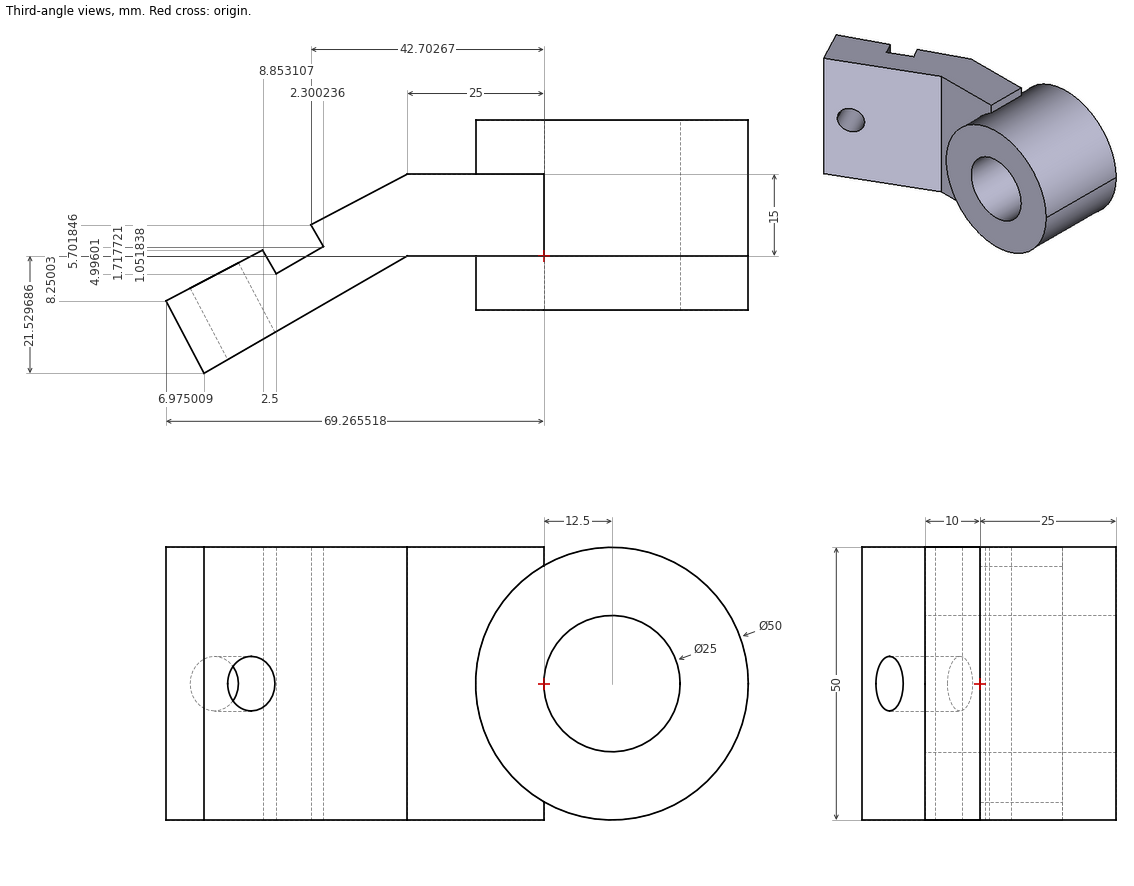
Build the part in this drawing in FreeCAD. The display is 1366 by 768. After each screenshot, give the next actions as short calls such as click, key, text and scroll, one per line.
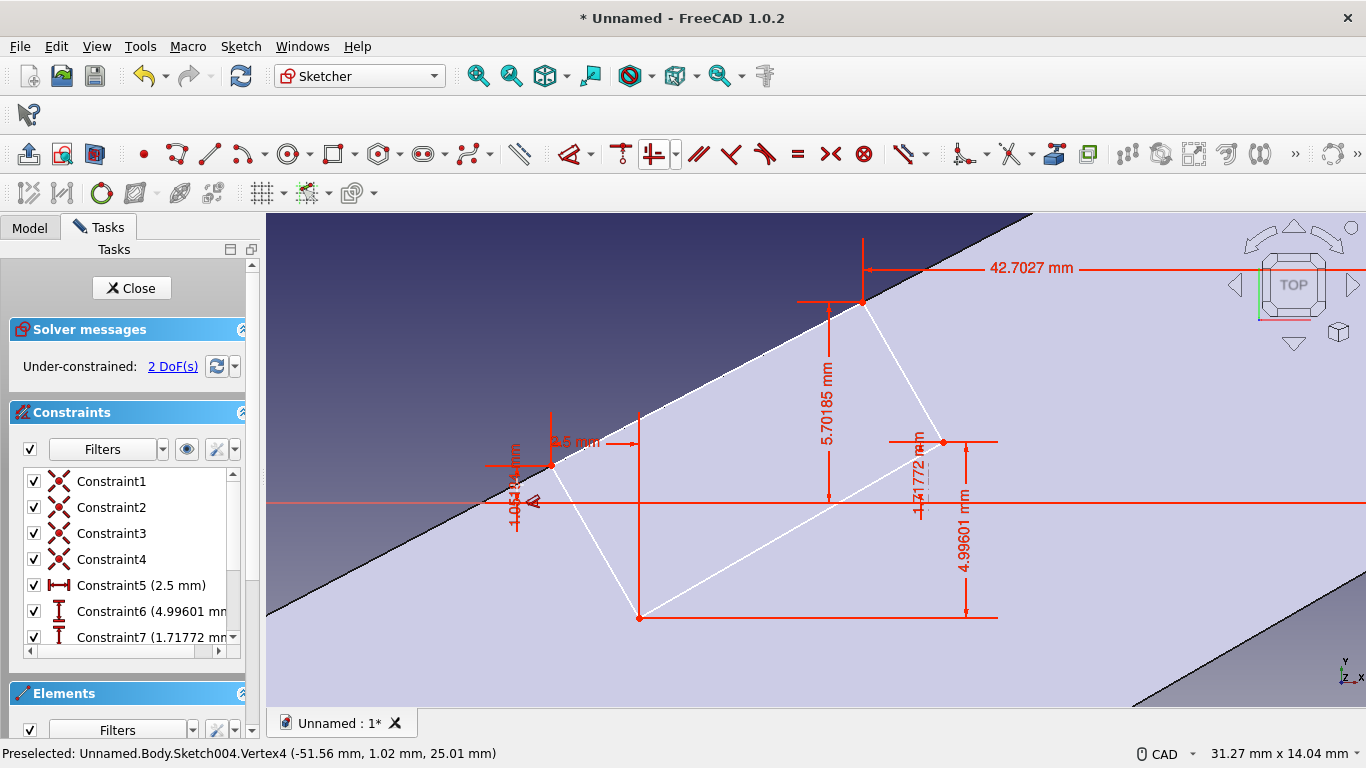
click(919, 400)
click(903, 268)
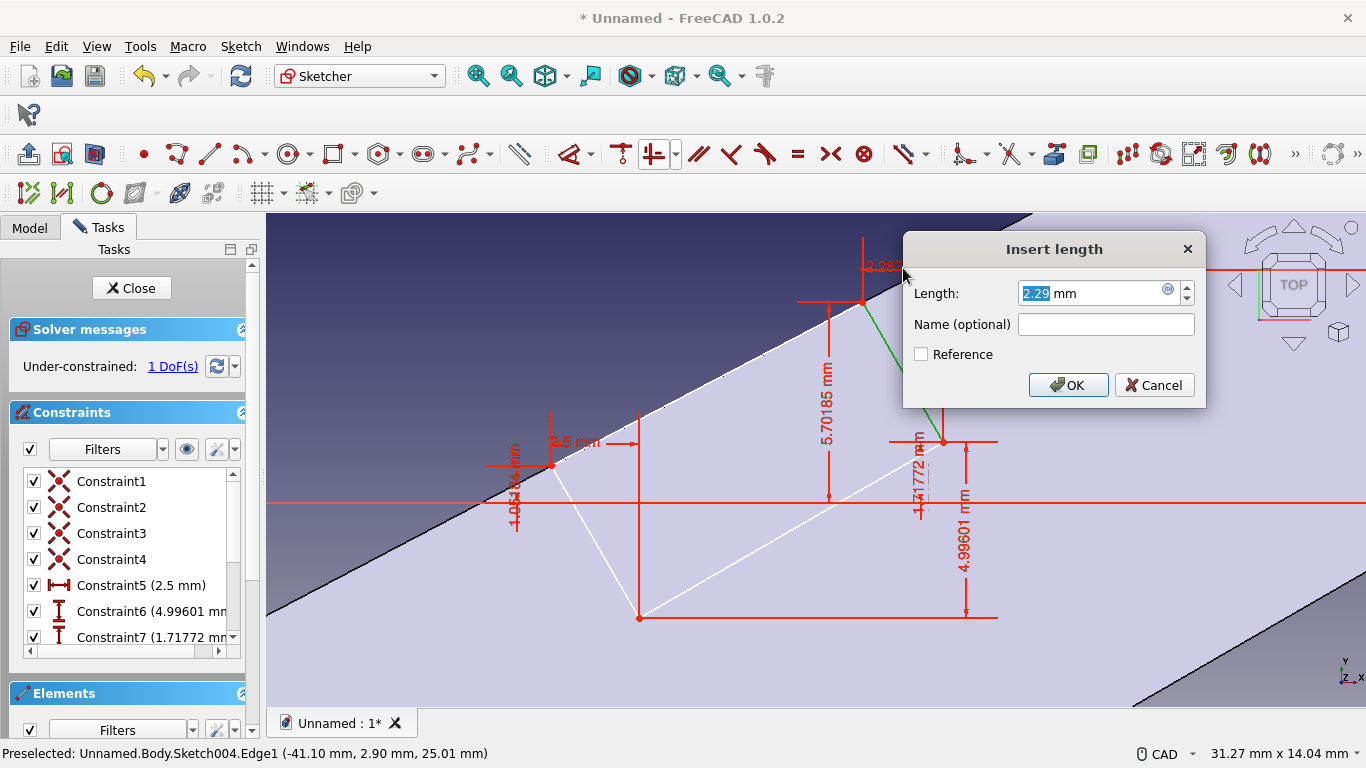
text(2.300236)
key(Return)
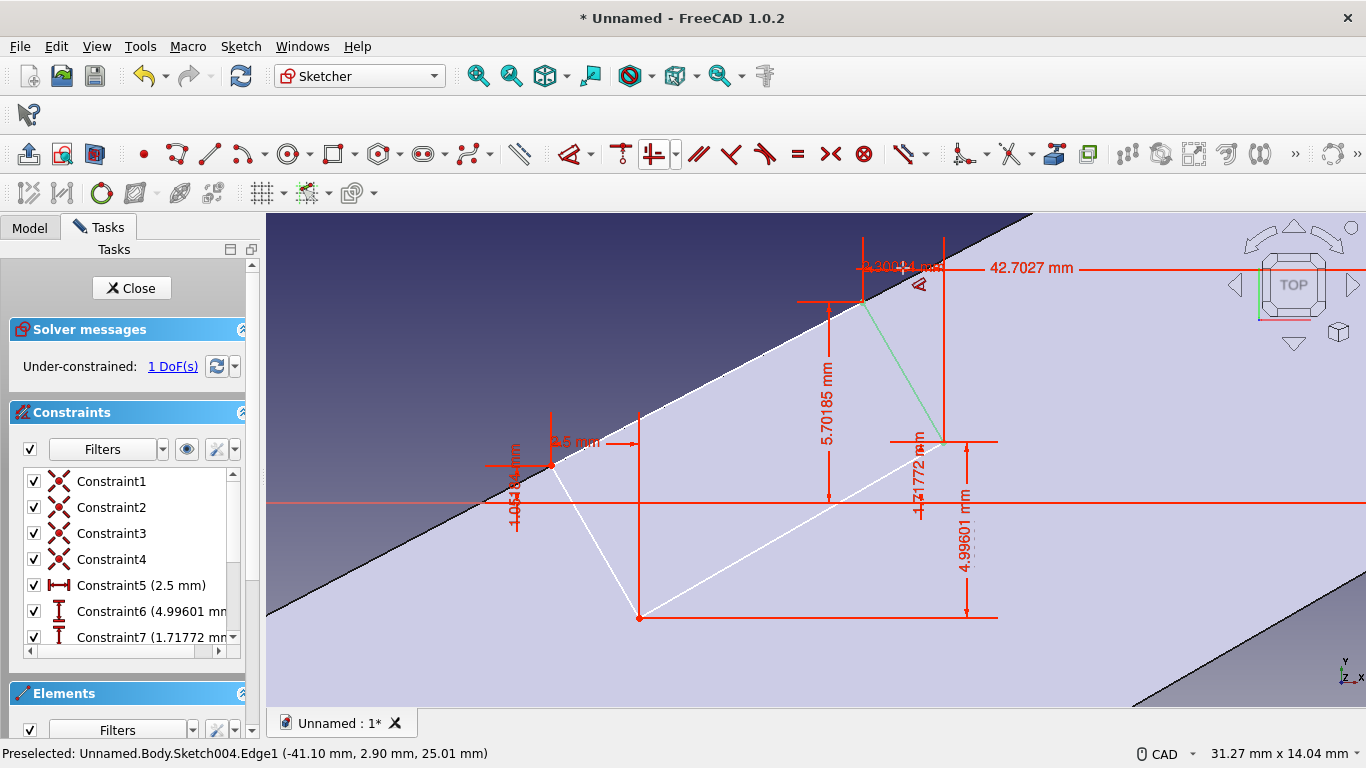
click(769, 351)
click(707, 268)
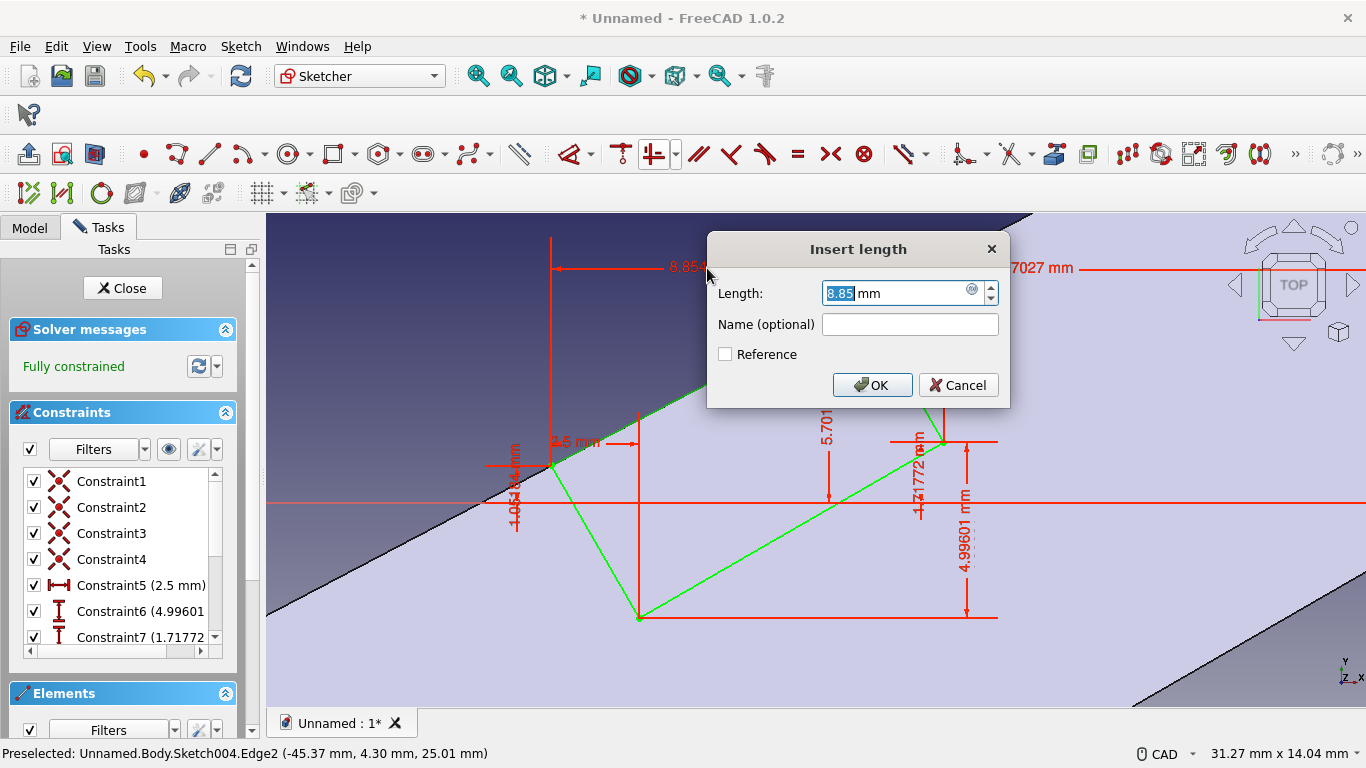
text(8.853107)
key(Return)
key(Escape)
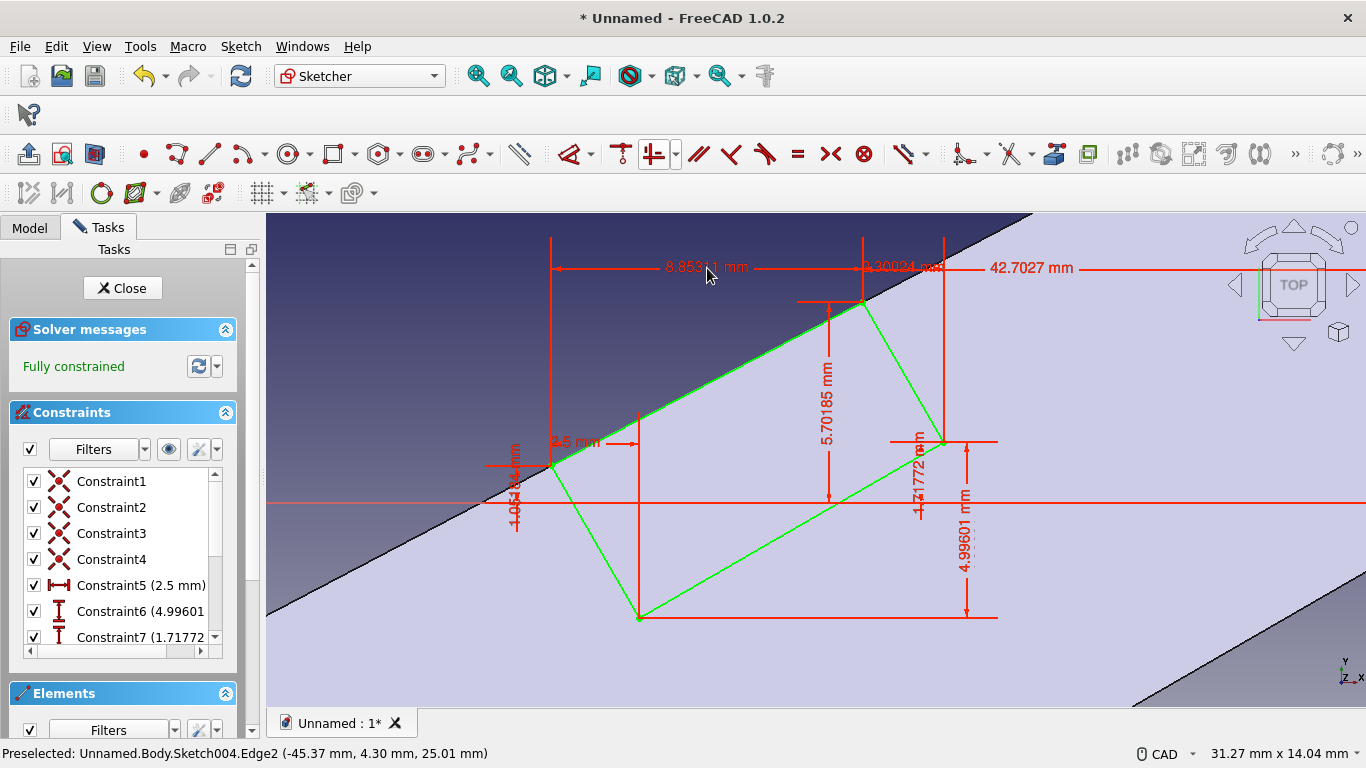
click(123, 288)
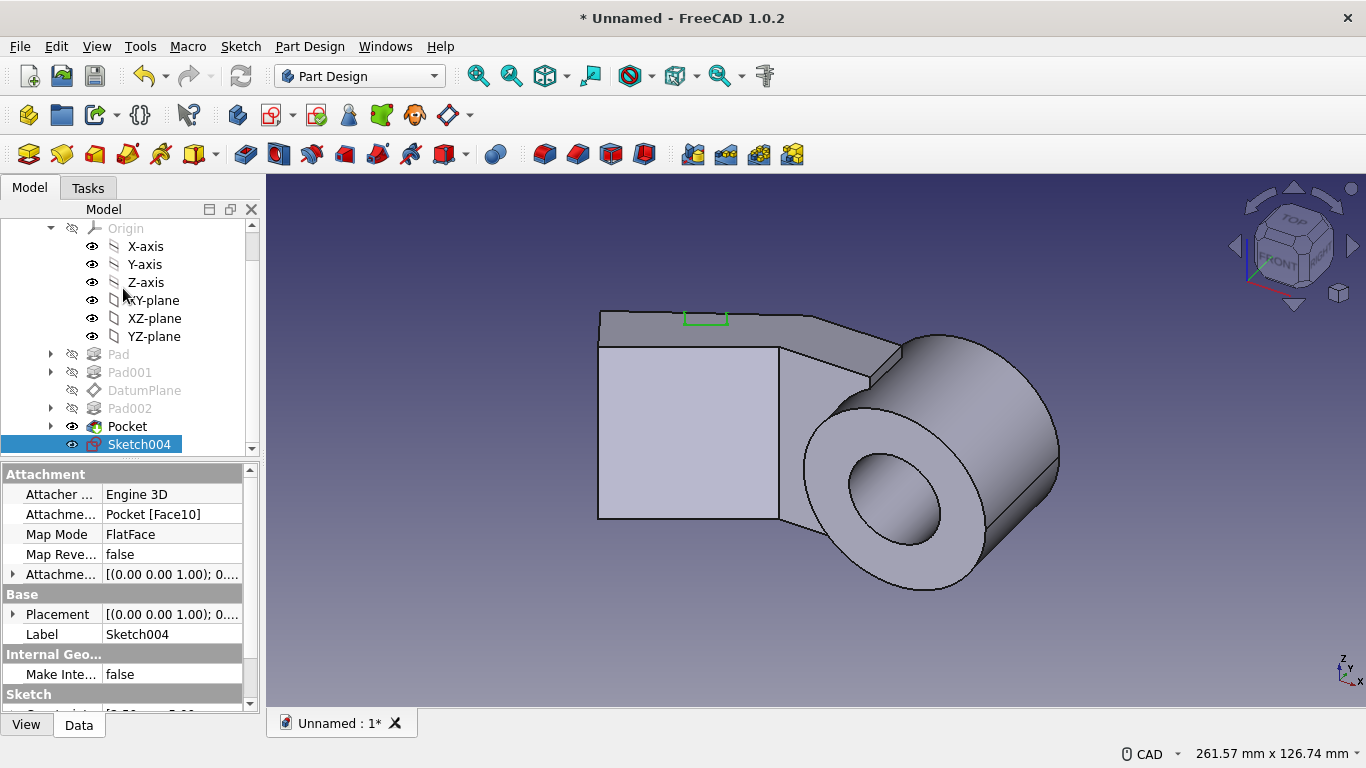
click(246, 154)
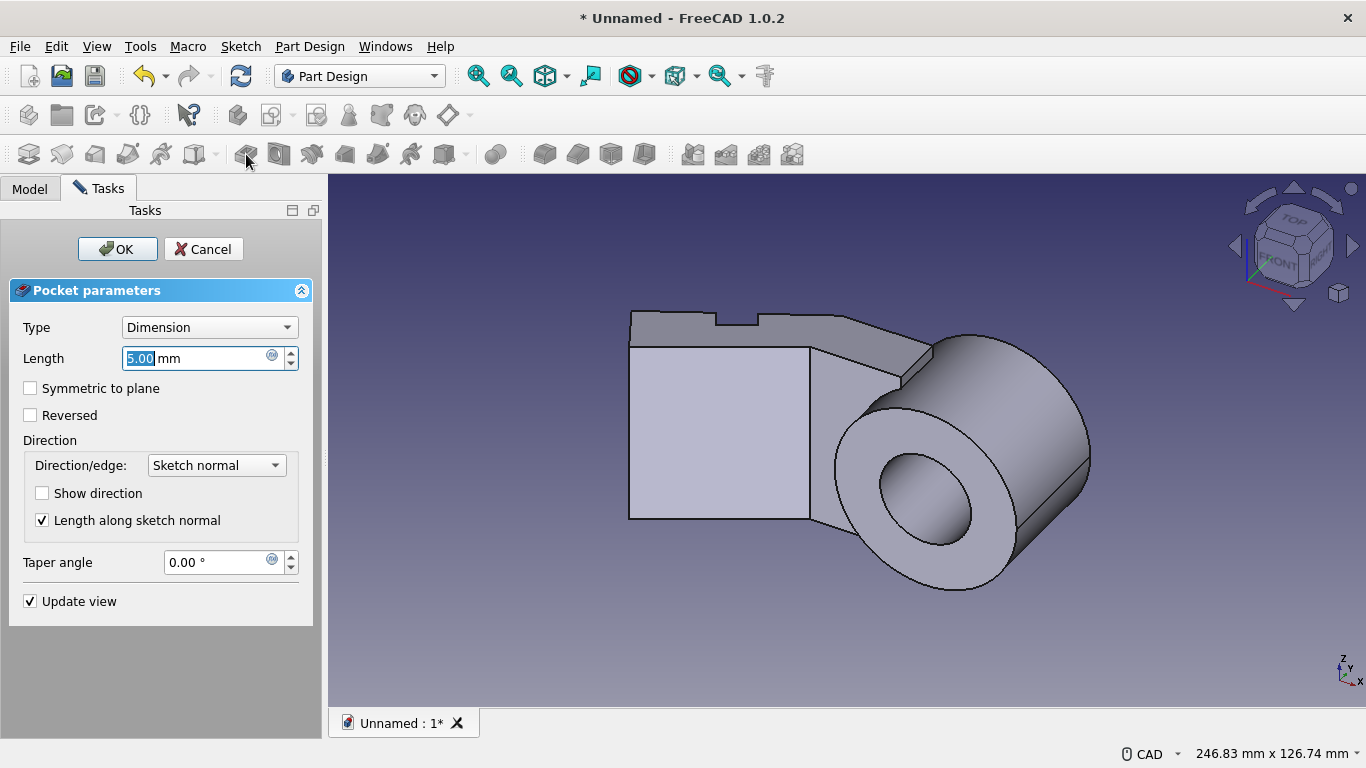
click(210, 328)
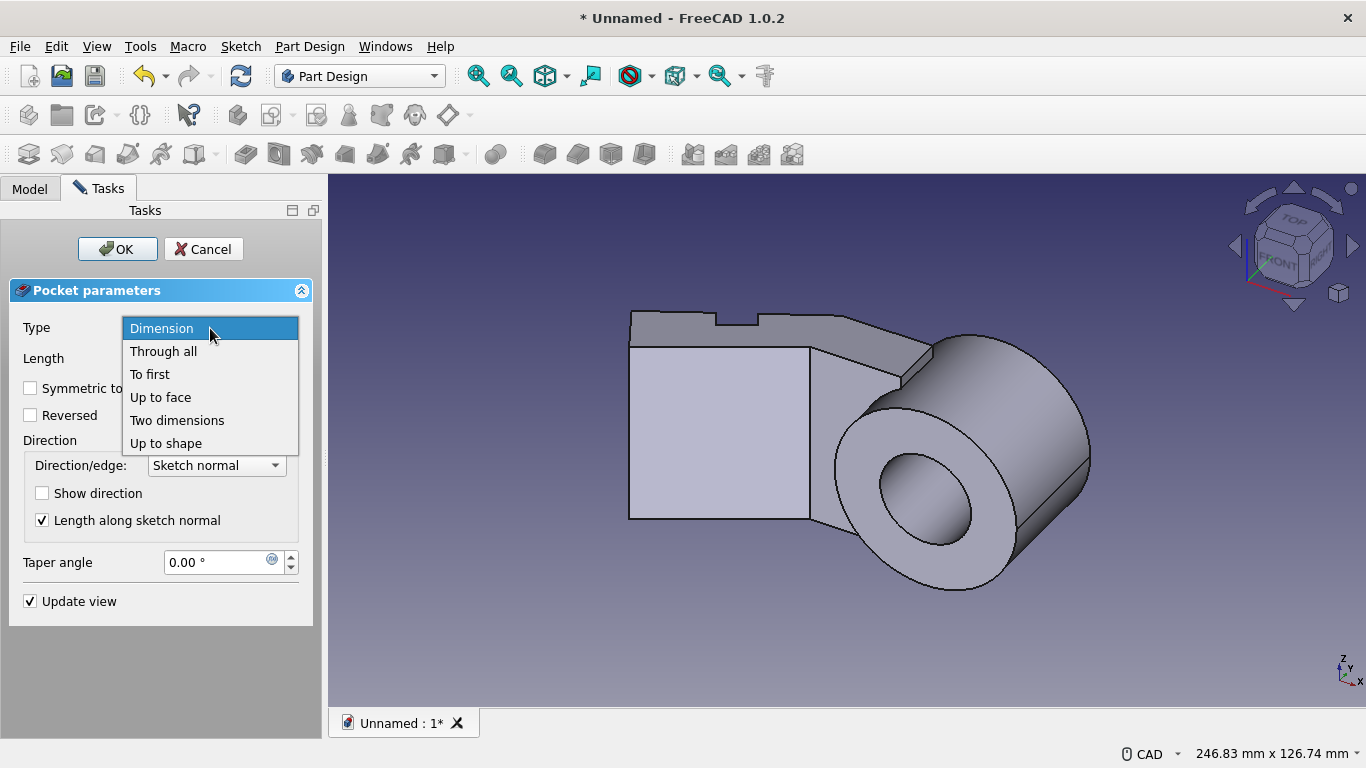
click(208, 352)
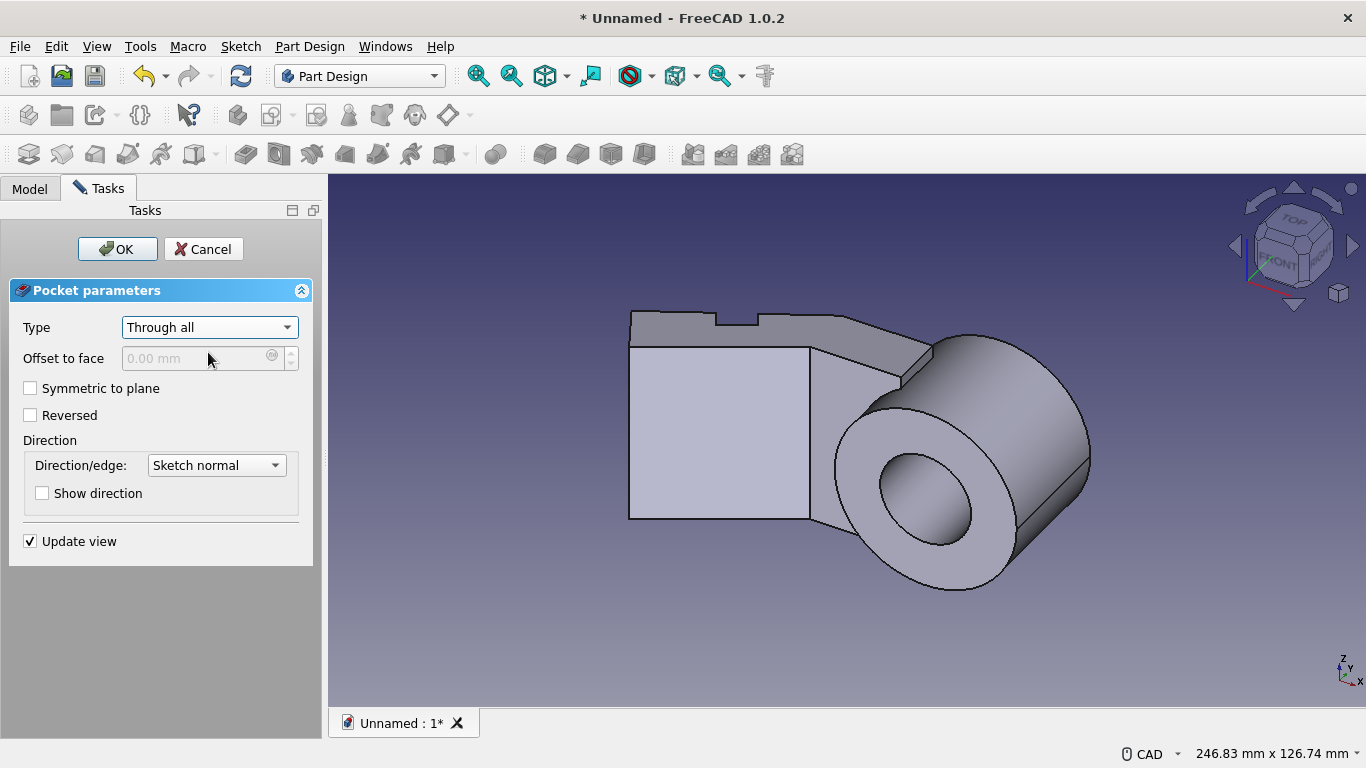
click(118, 249)